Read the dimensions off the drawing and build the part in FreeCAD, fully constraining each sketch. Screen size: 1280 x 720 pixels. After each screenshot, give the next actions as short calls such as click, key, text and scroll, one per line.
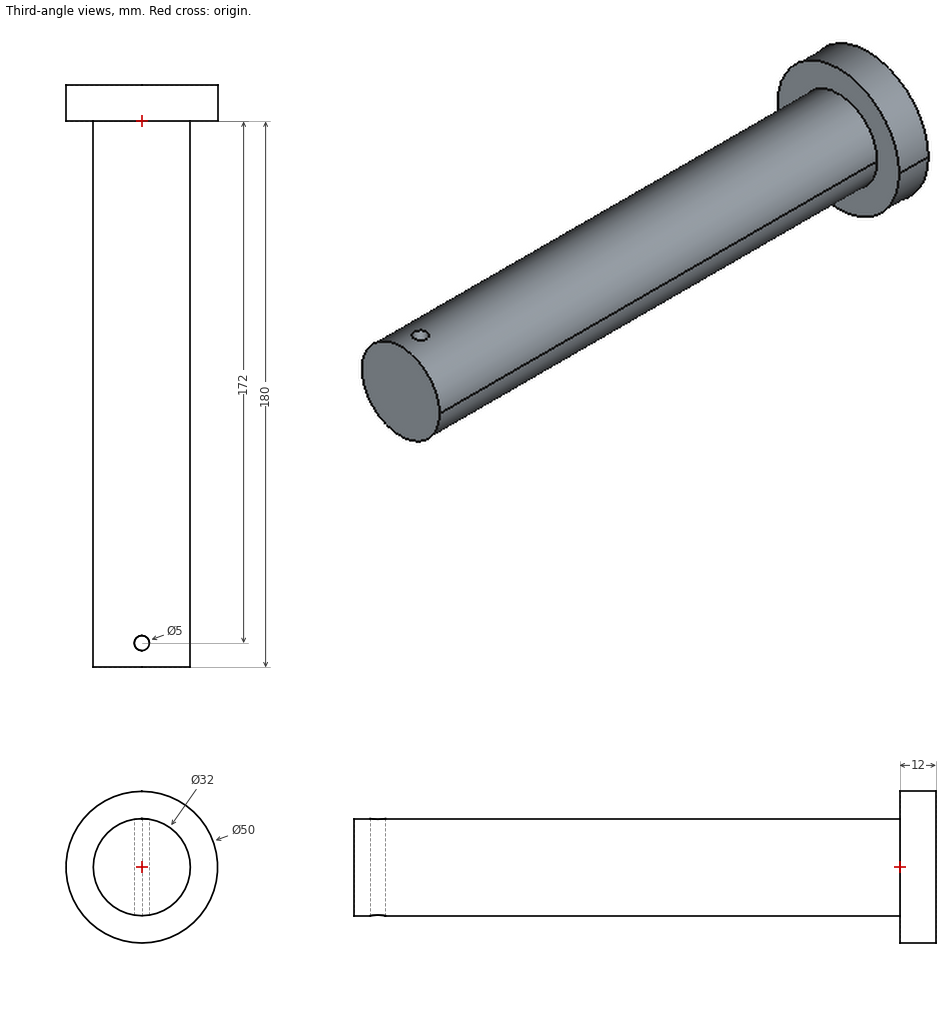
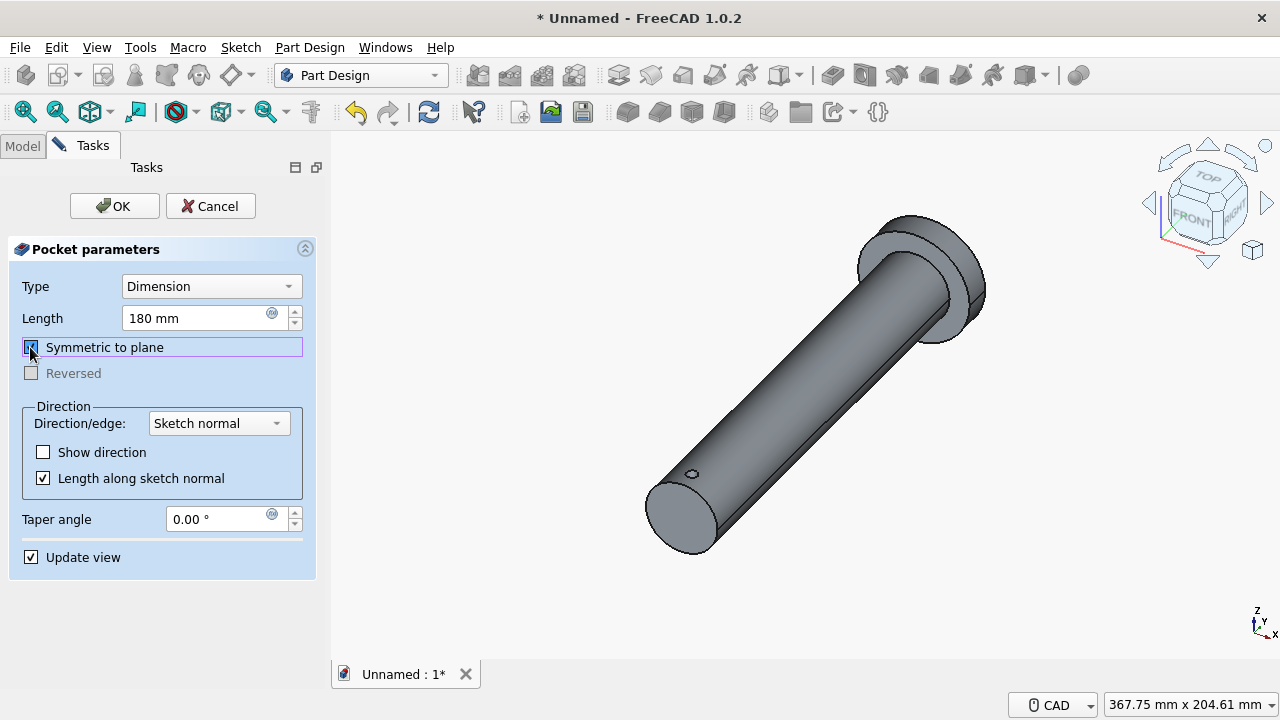
click(115, 206)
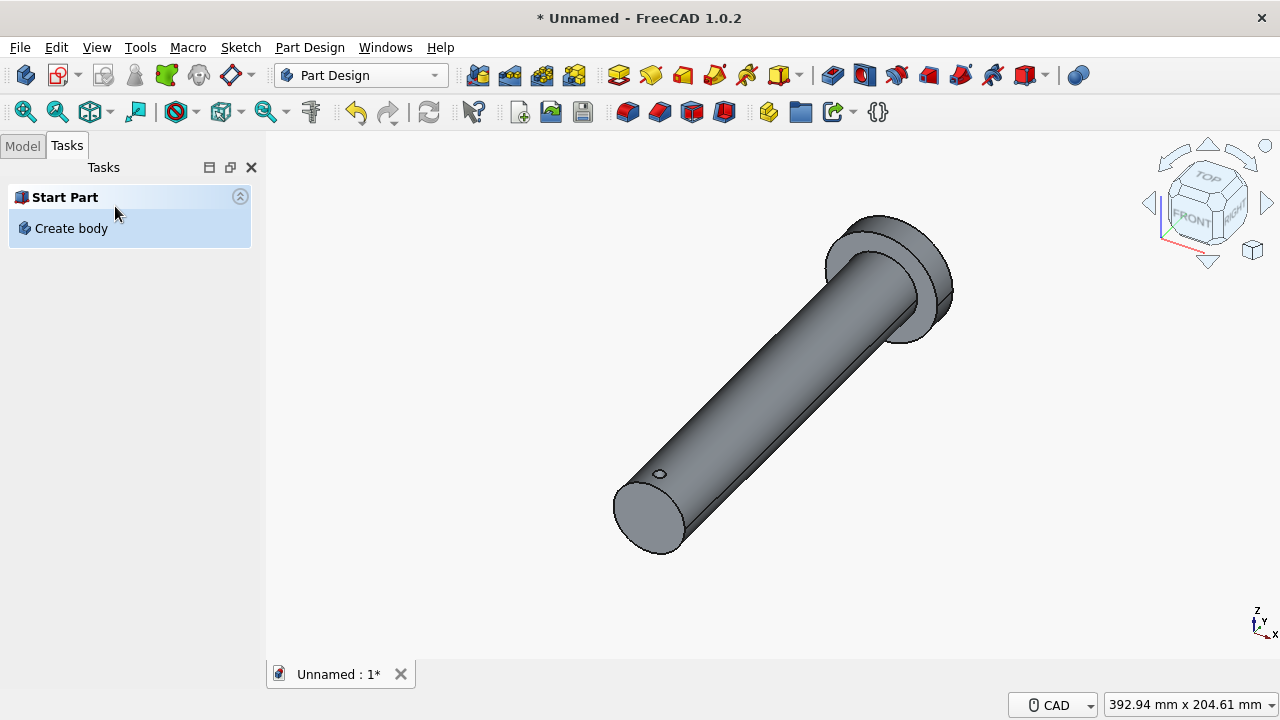
key(0)